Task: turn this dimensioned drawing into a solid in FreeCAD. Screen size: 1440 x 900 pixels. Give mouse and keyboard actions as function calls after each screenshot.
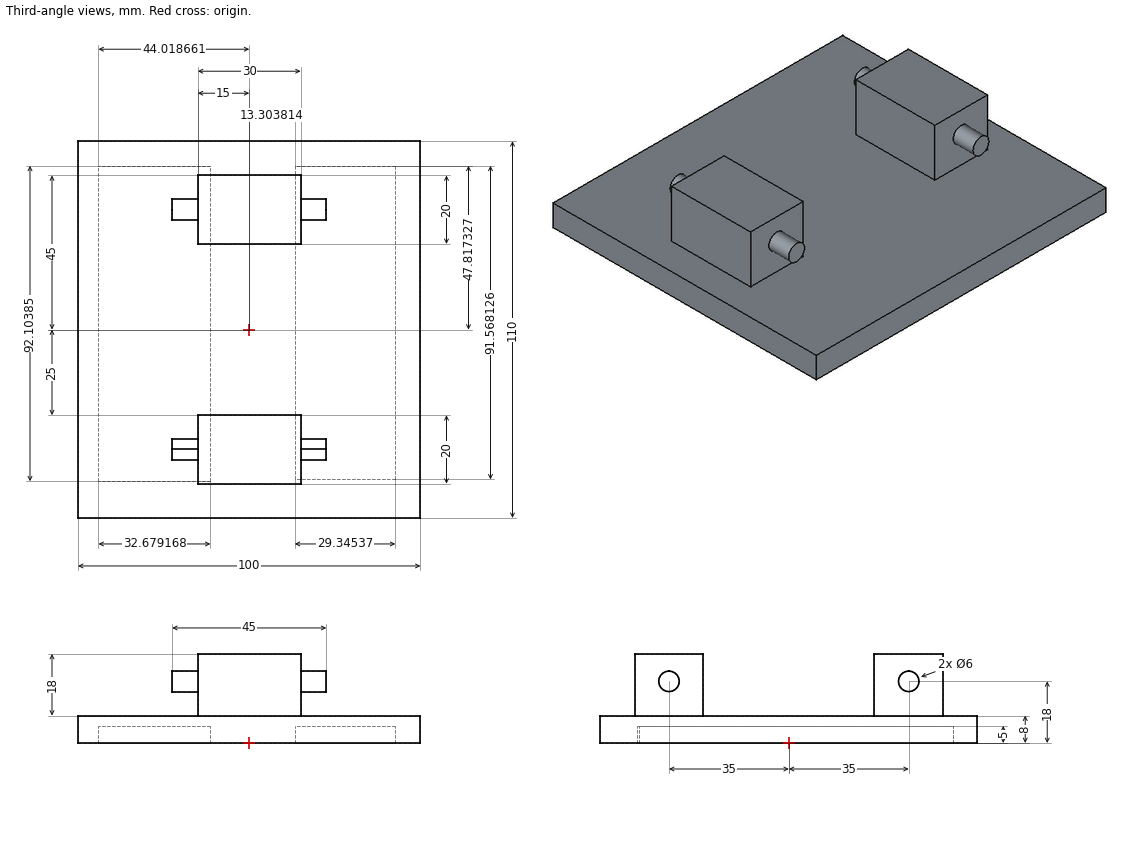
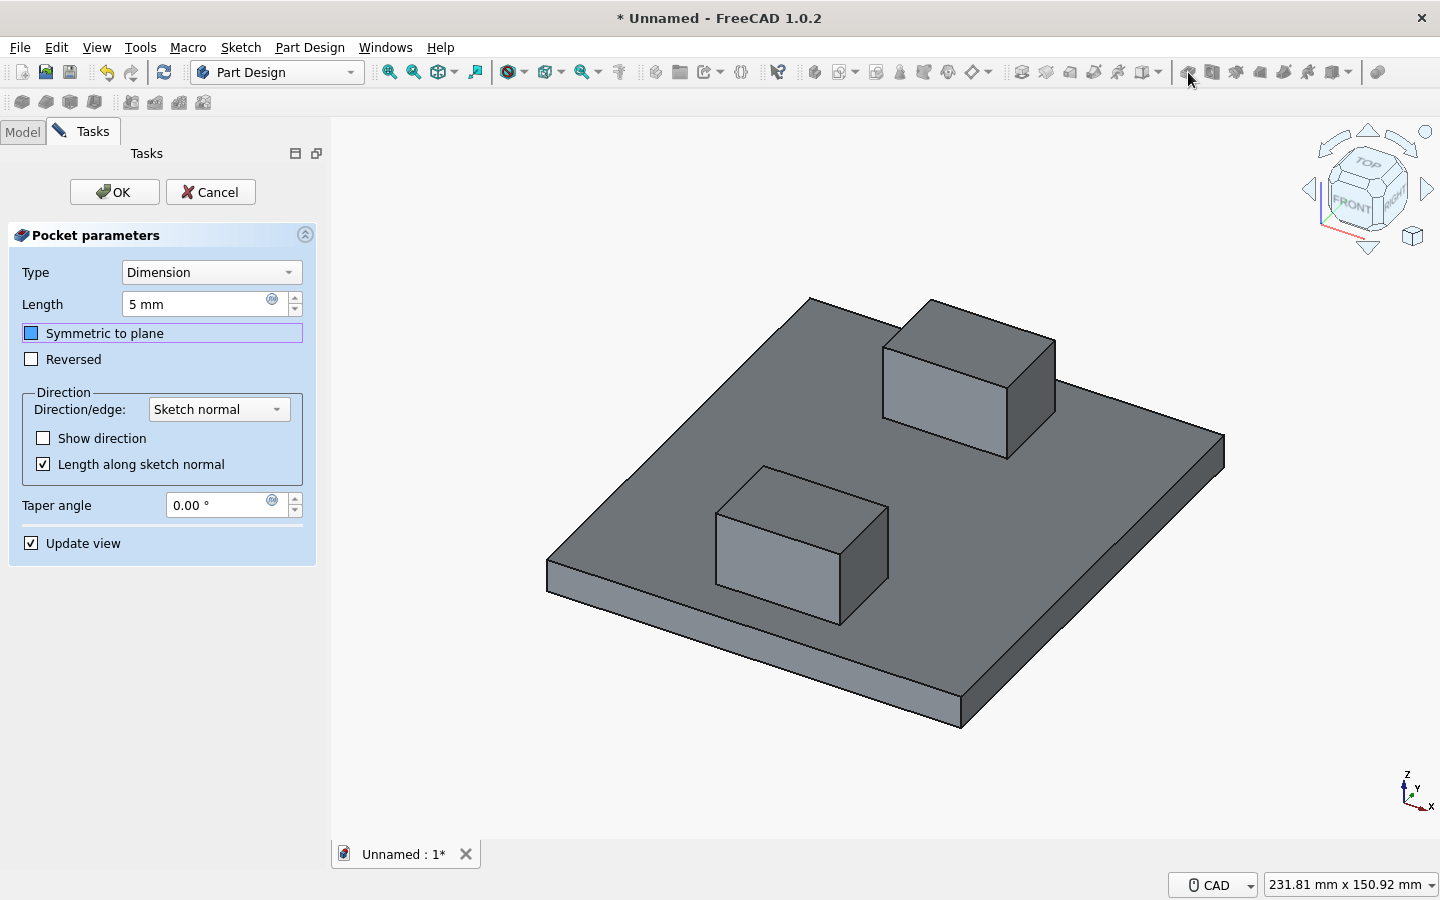
click(30, 359)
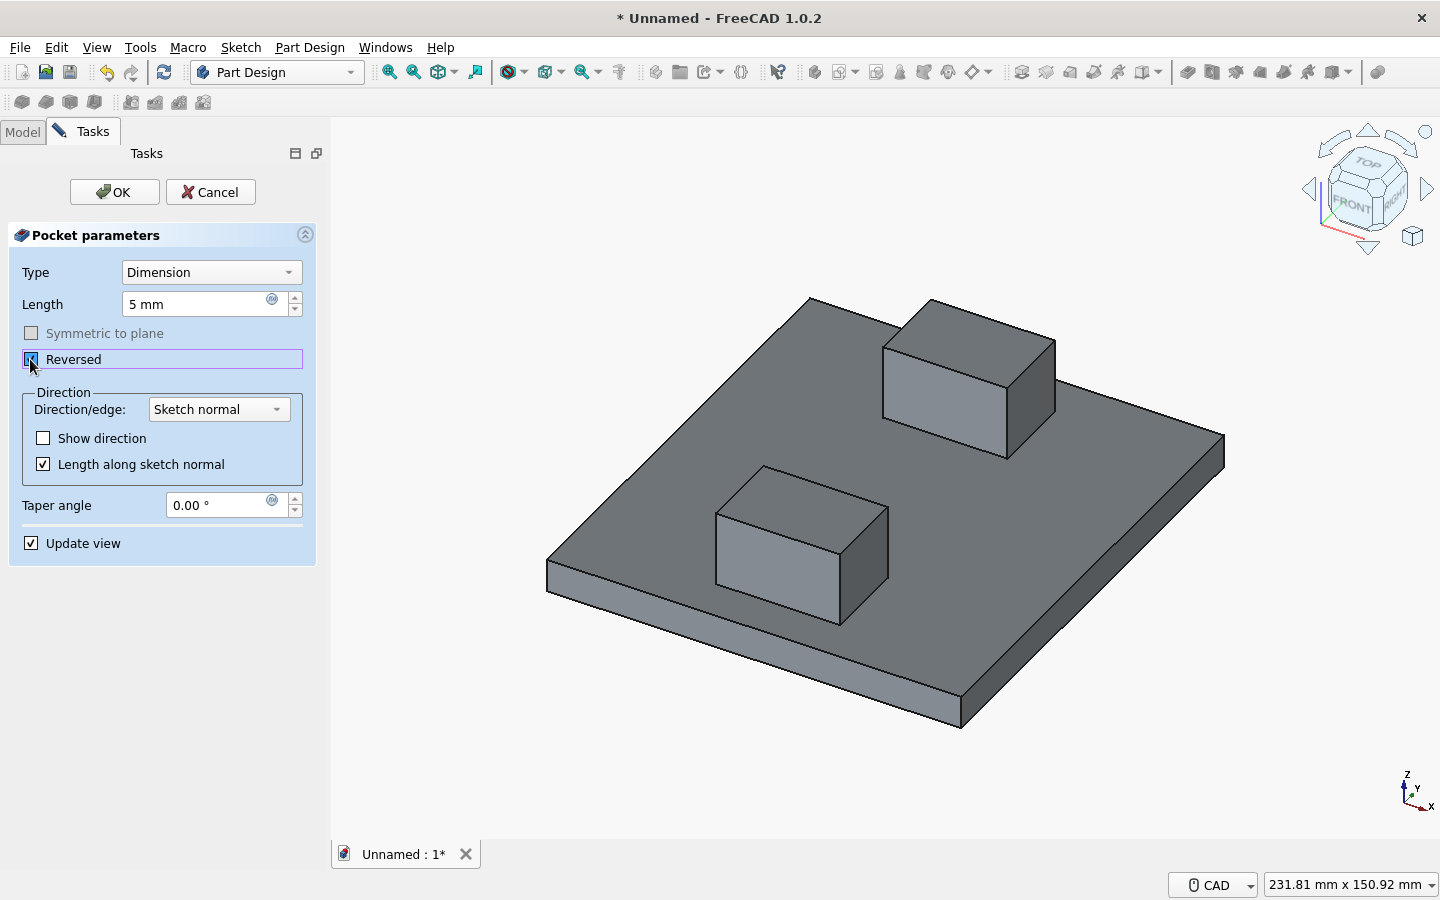
click(115, 192)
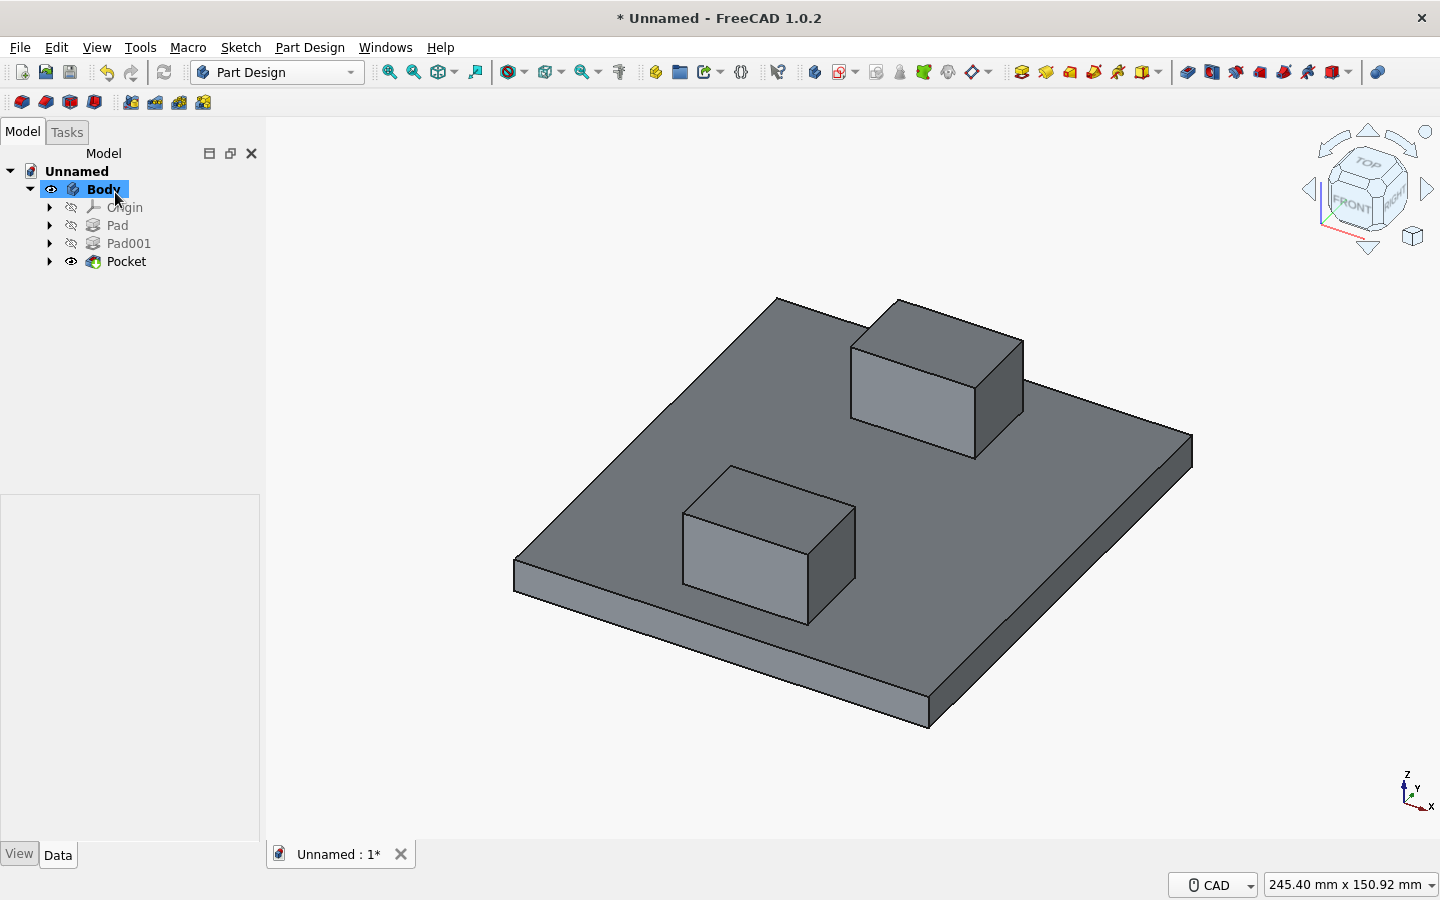
click(840, 72)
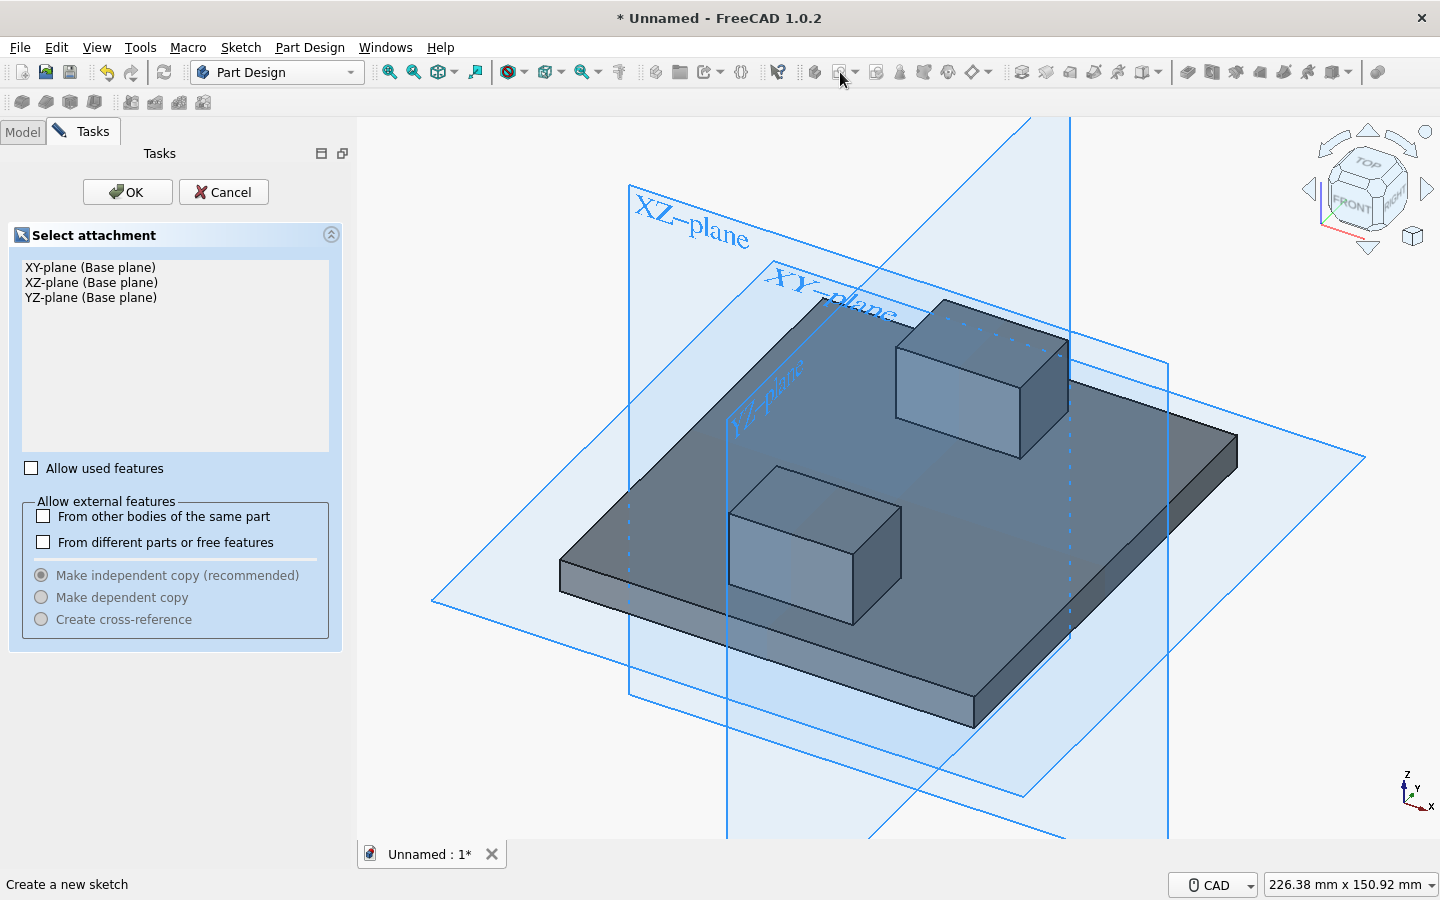
click(82, 298)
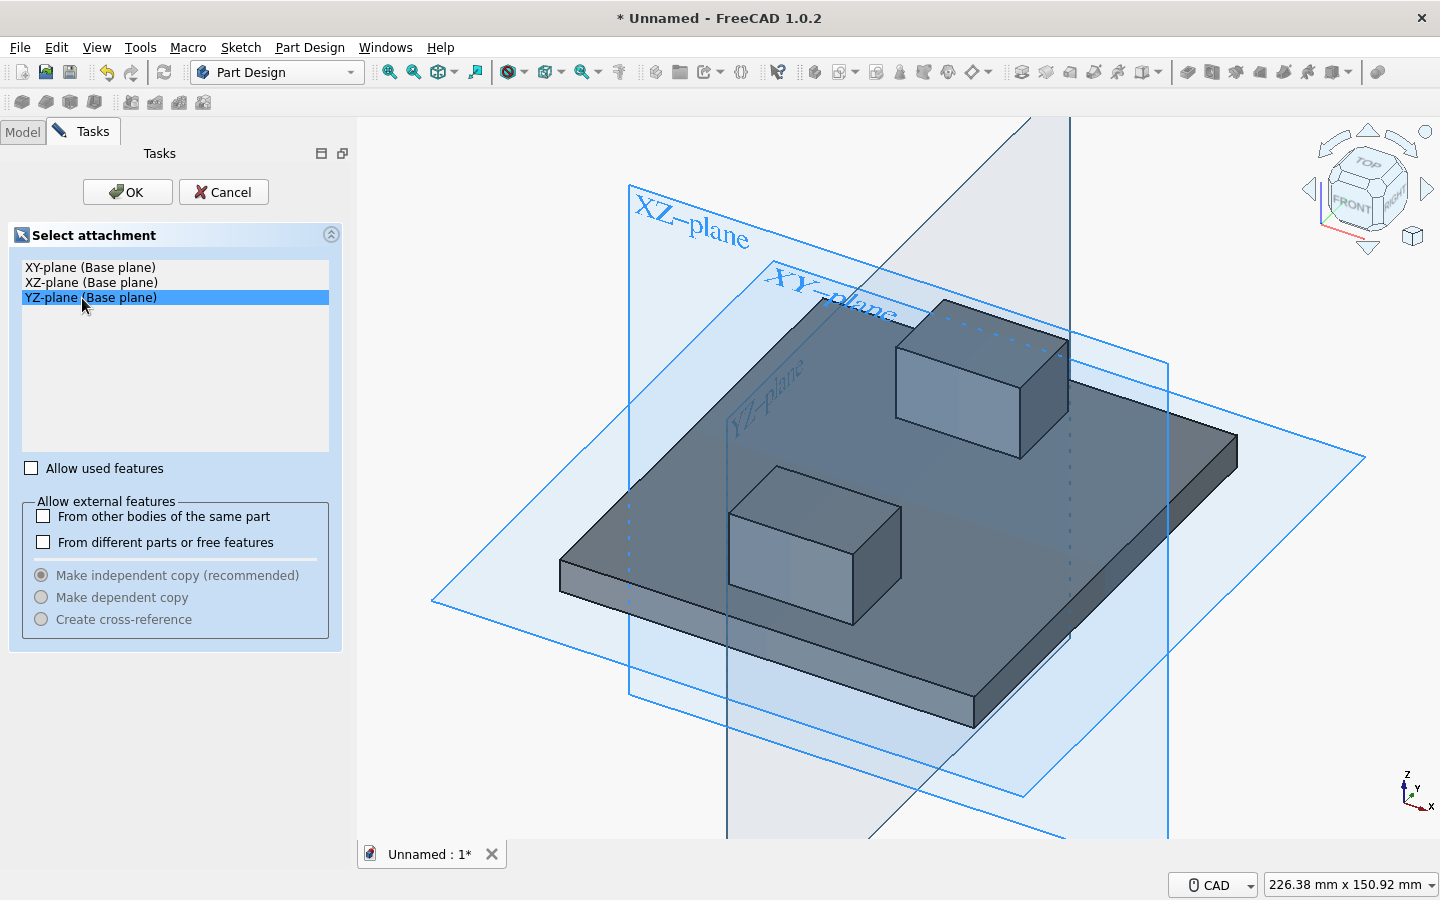
click(128, 192)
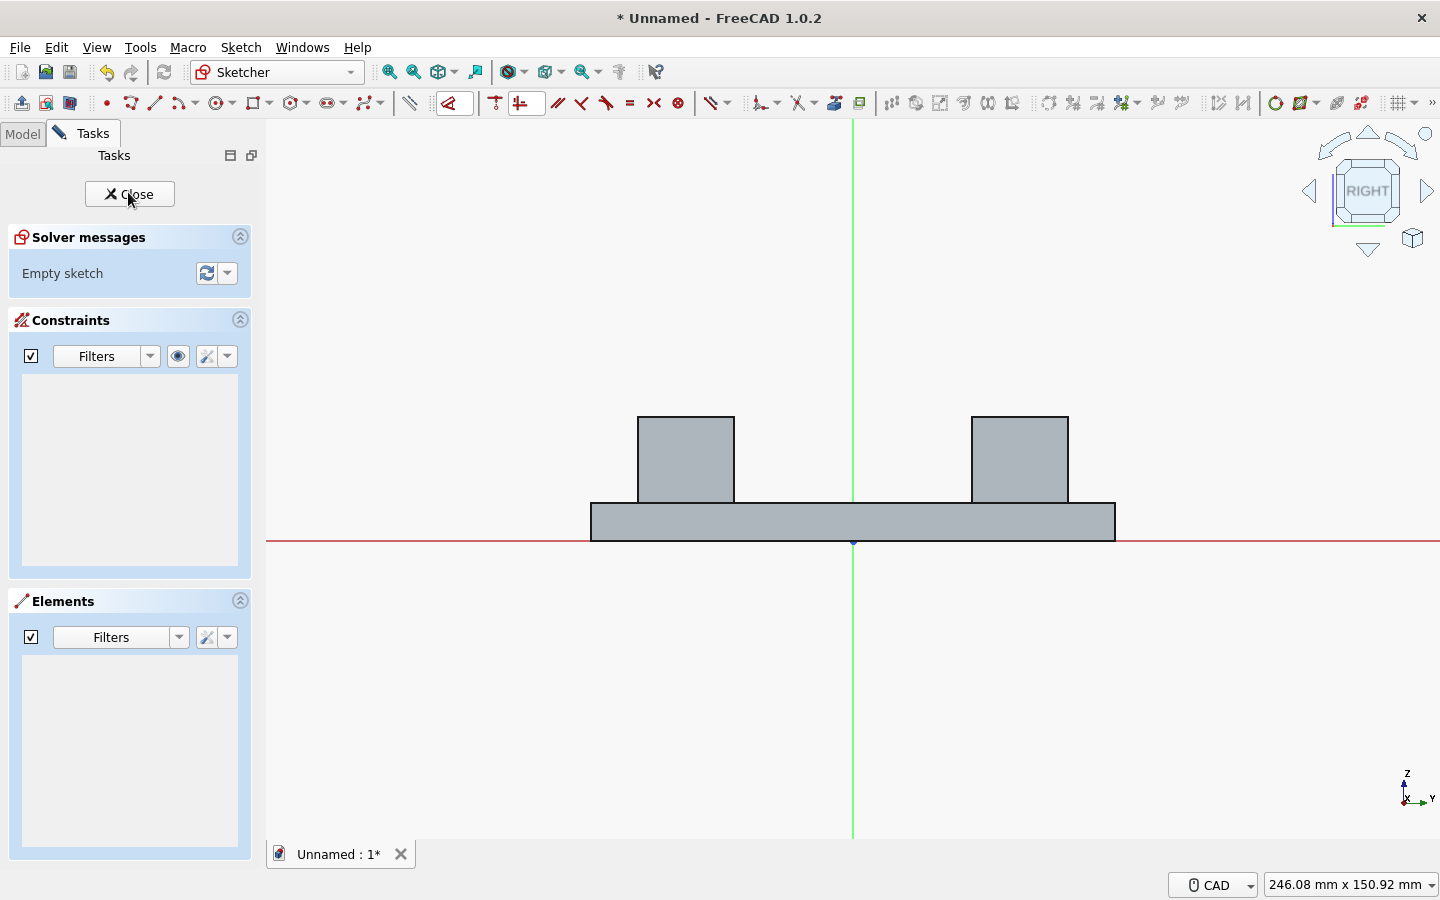
click(70, 104)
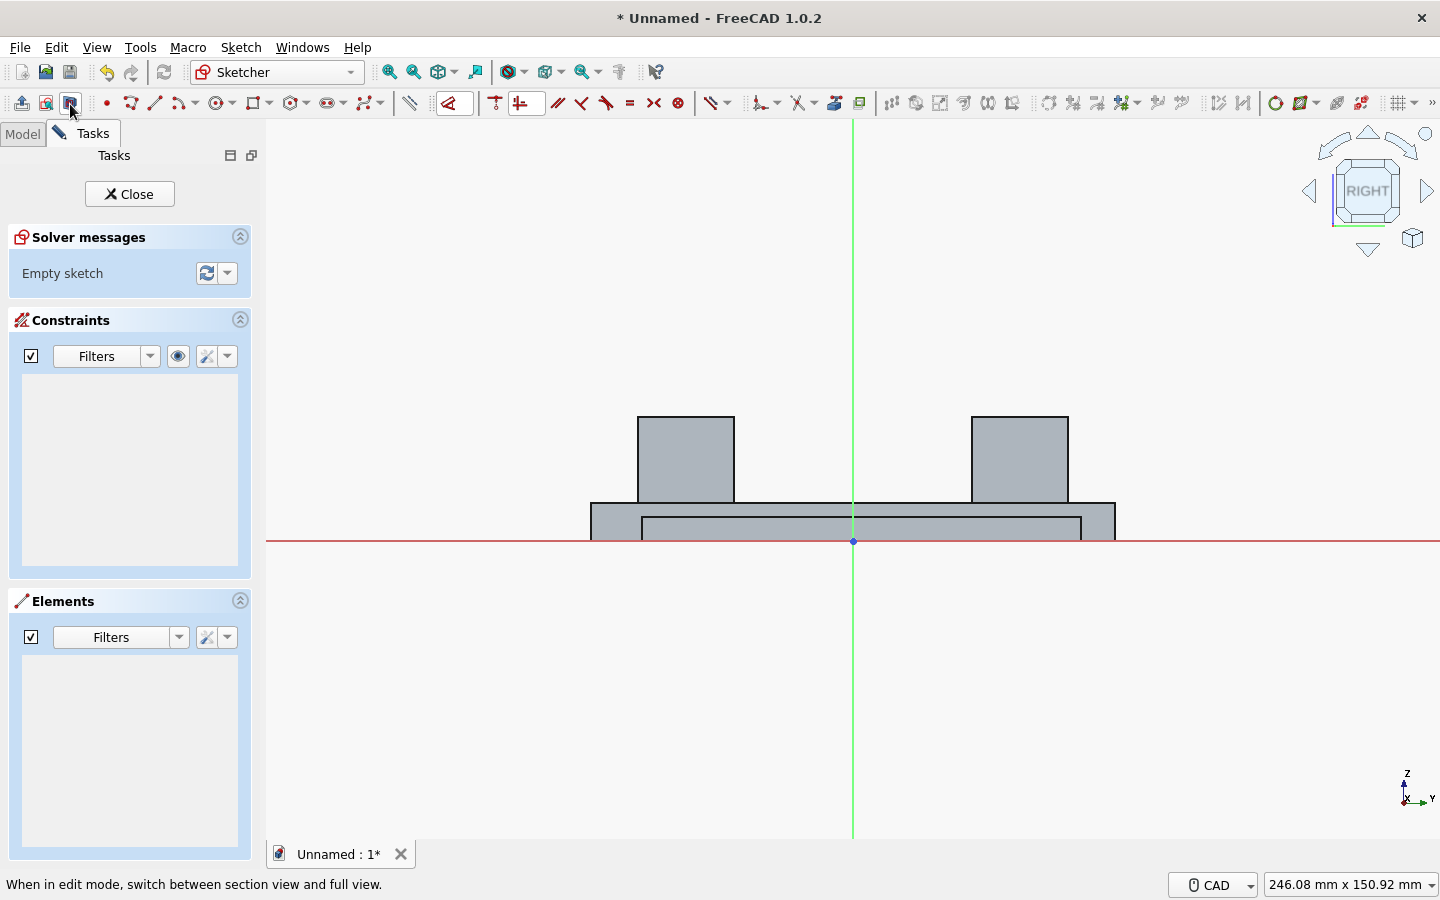
scroll(936, 505, up, 3)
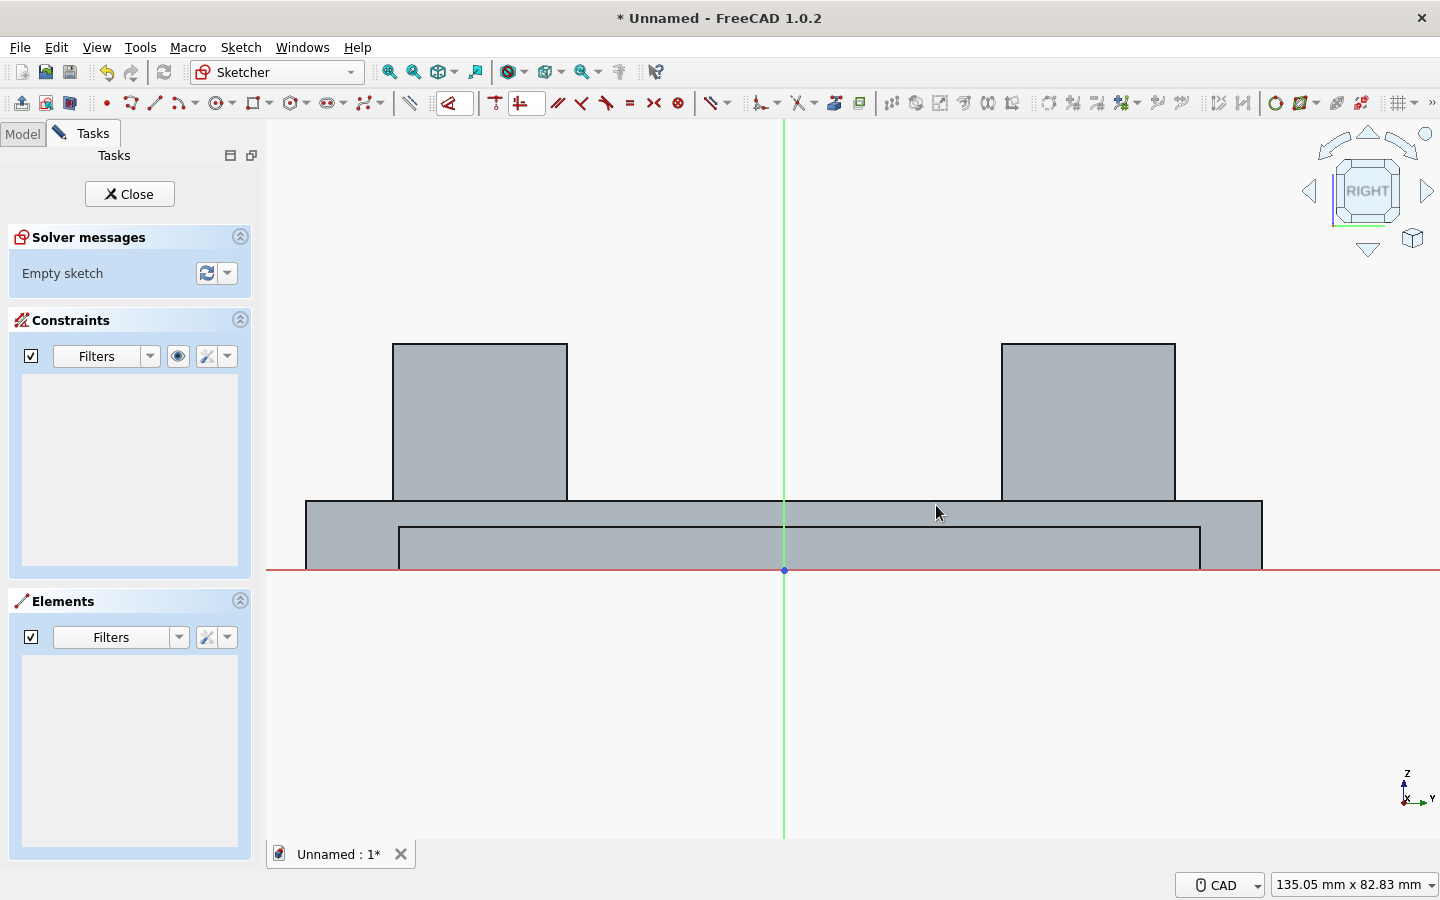
key(g)
key(c)